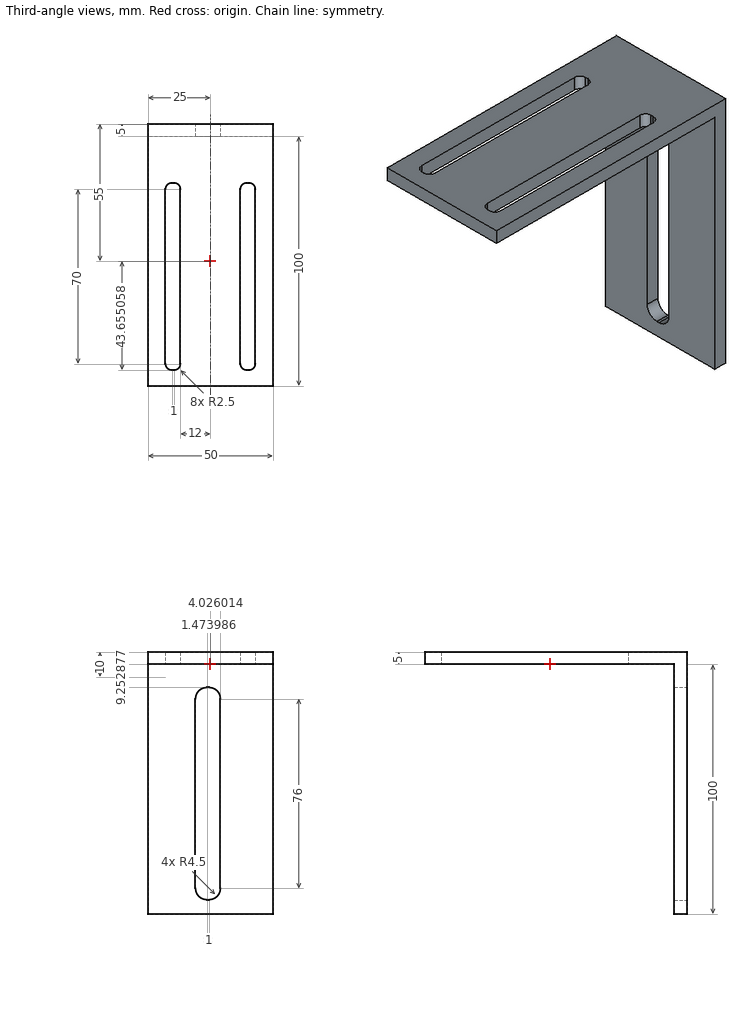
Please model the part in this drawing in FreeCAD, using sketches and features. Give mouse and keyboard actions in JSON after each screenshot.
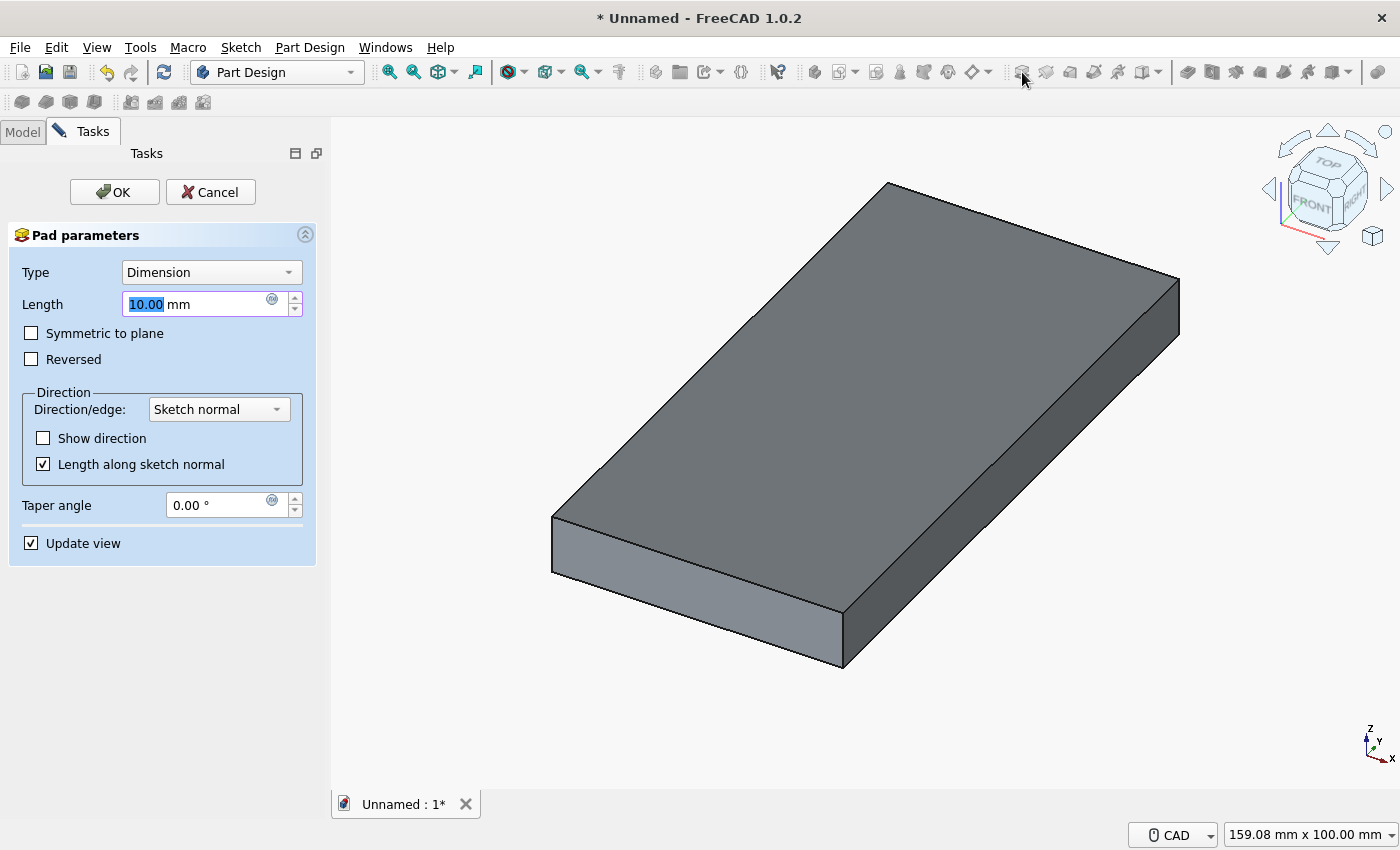
{"action": "type", "text": "5"}
{"action": "key", "text": "Tab"}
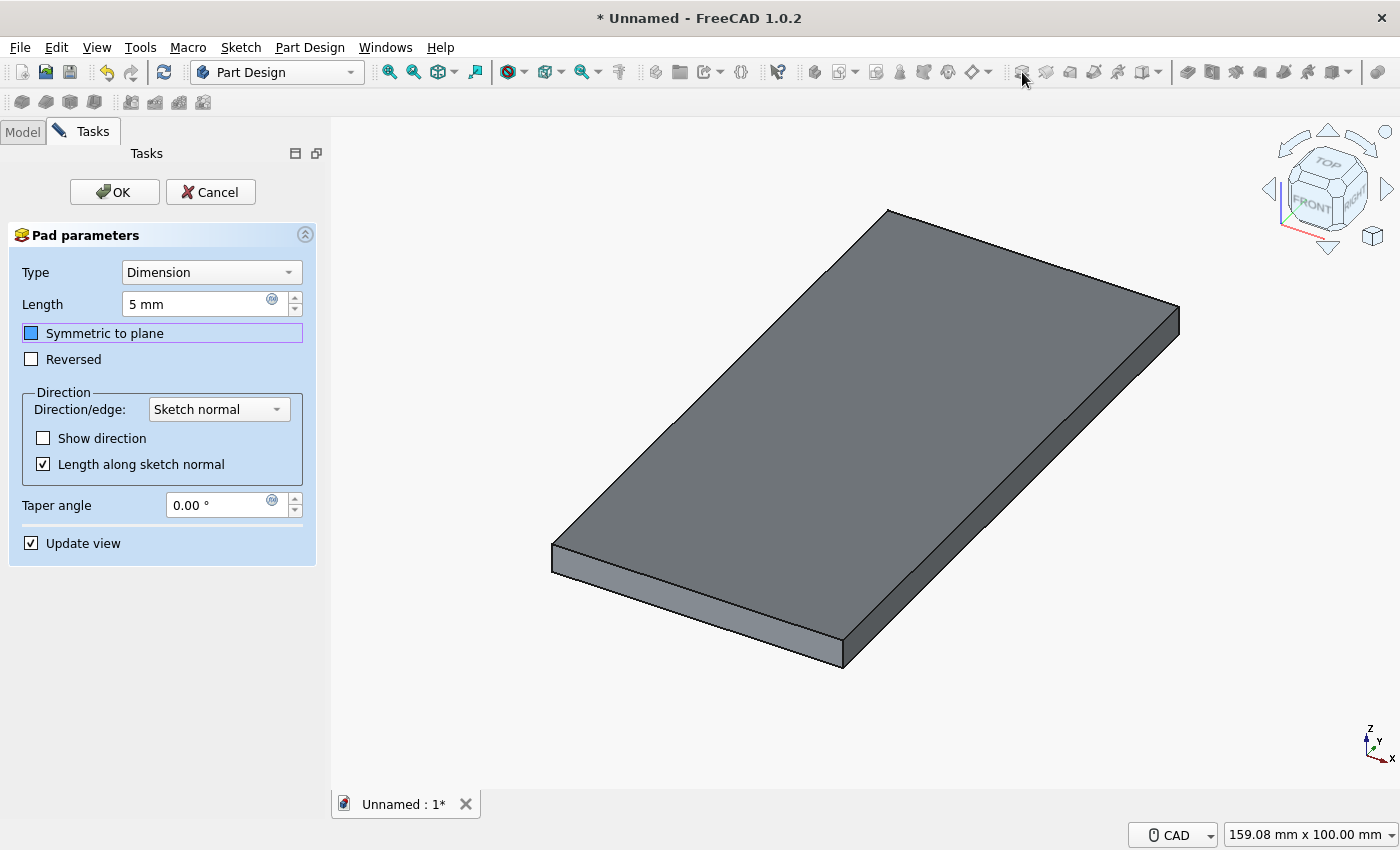
{"action": "left_click", "coordinate": [115, 192]}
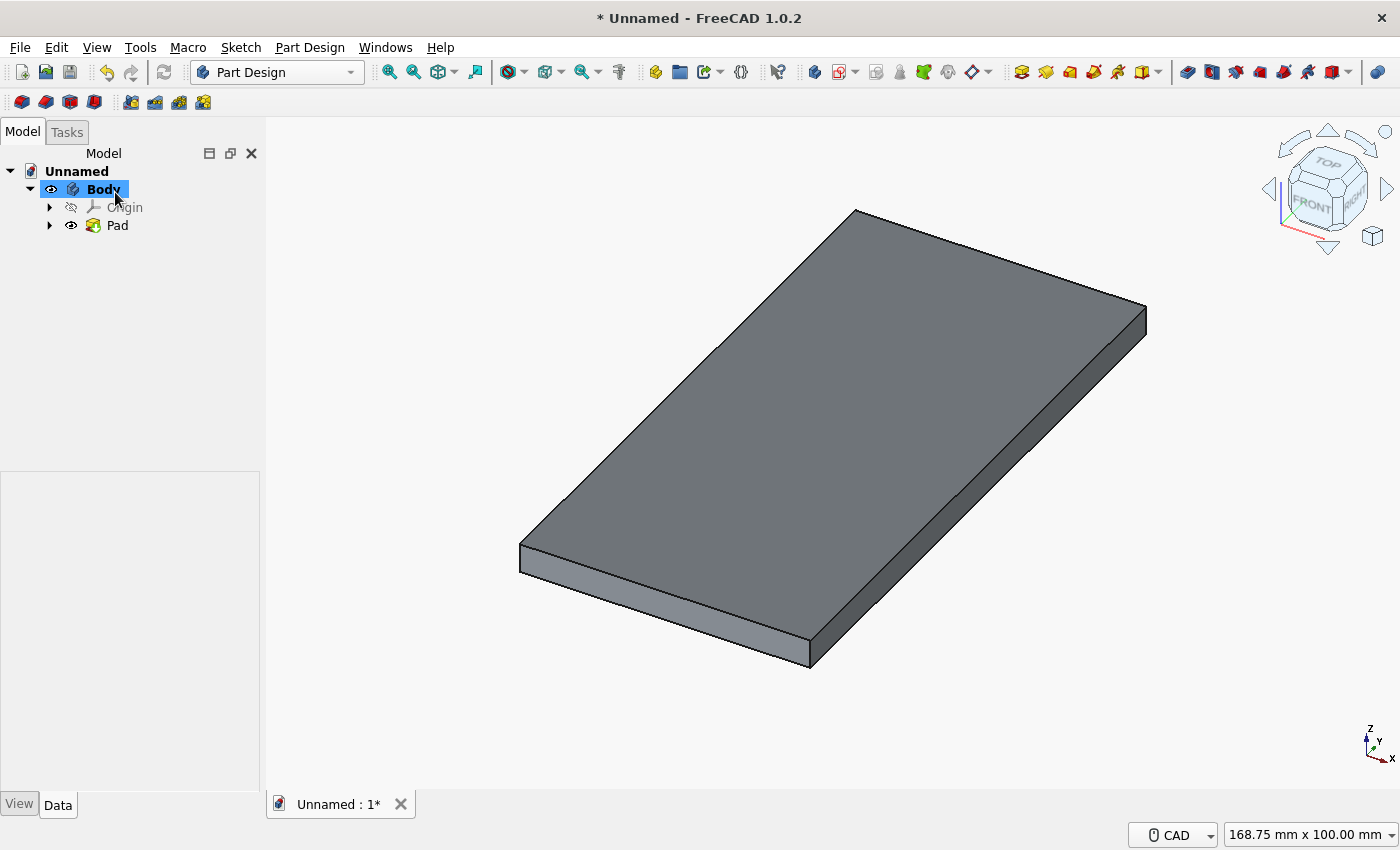
{"action": "left_click", "coordinate": [881, 377]}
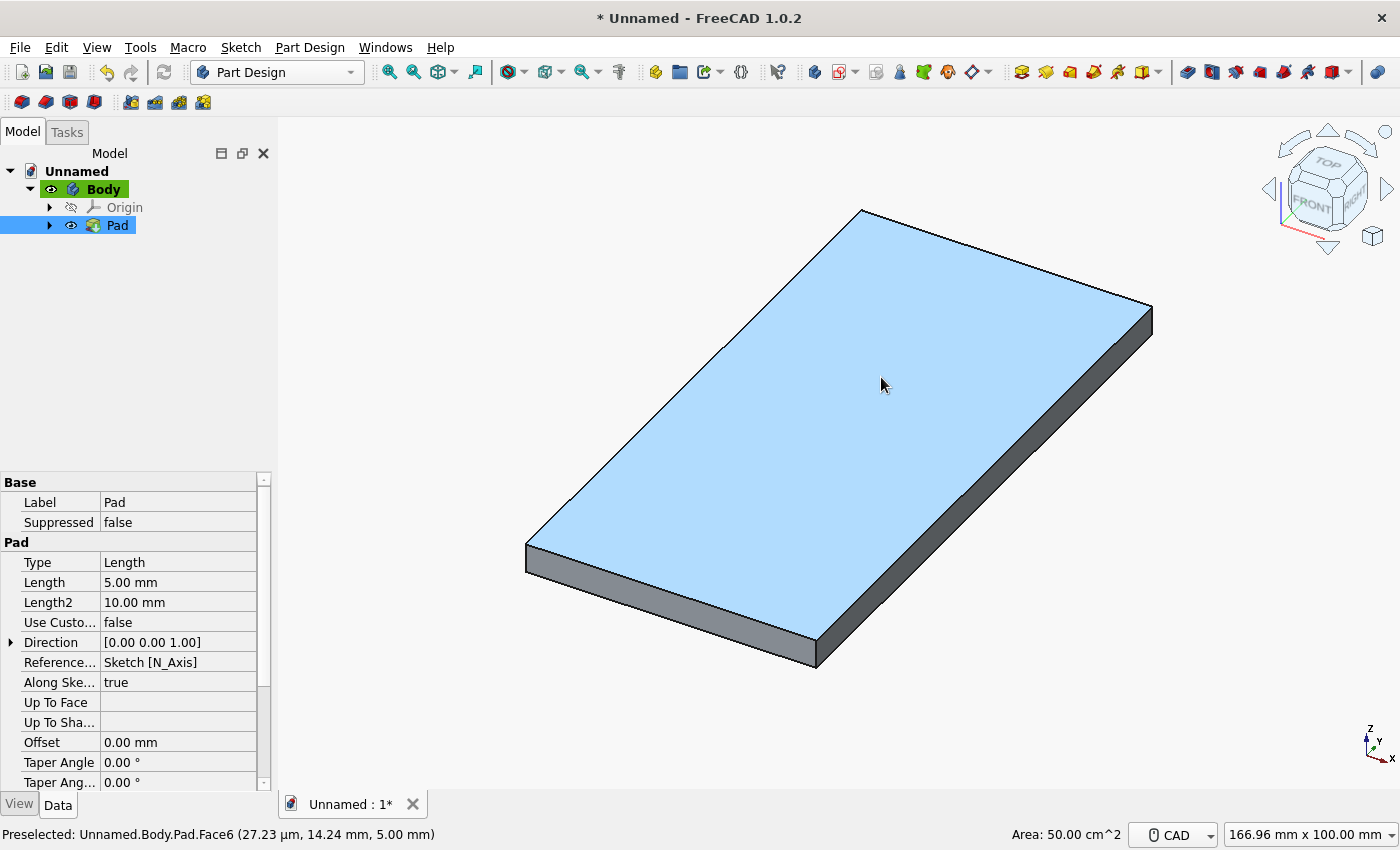
{"action": "left_click", "coordinate": [840, 72]}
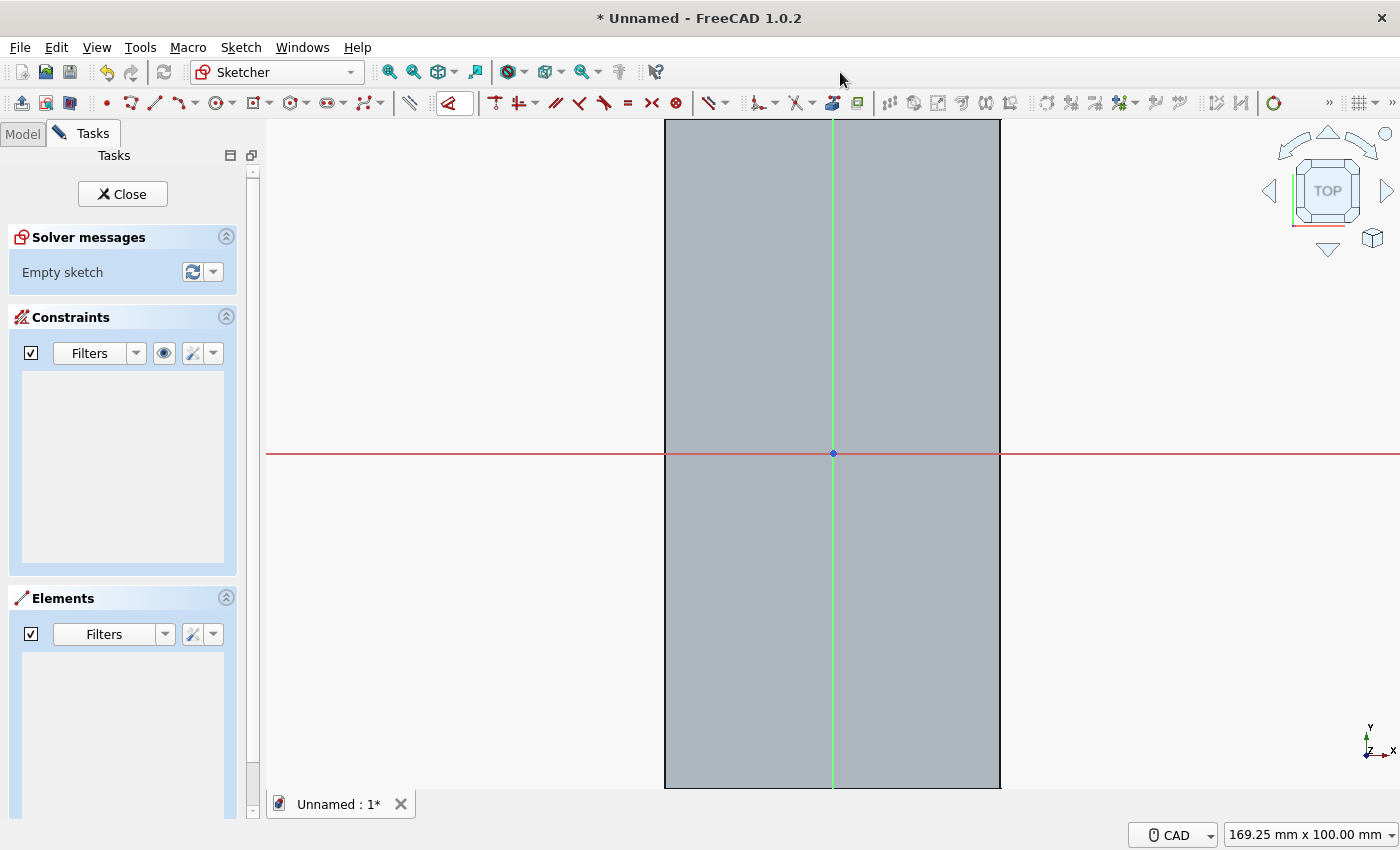
{"action": "scroll", "coordinate": [455, 268], "scroll_direction": "down", "scroll_amount": 1}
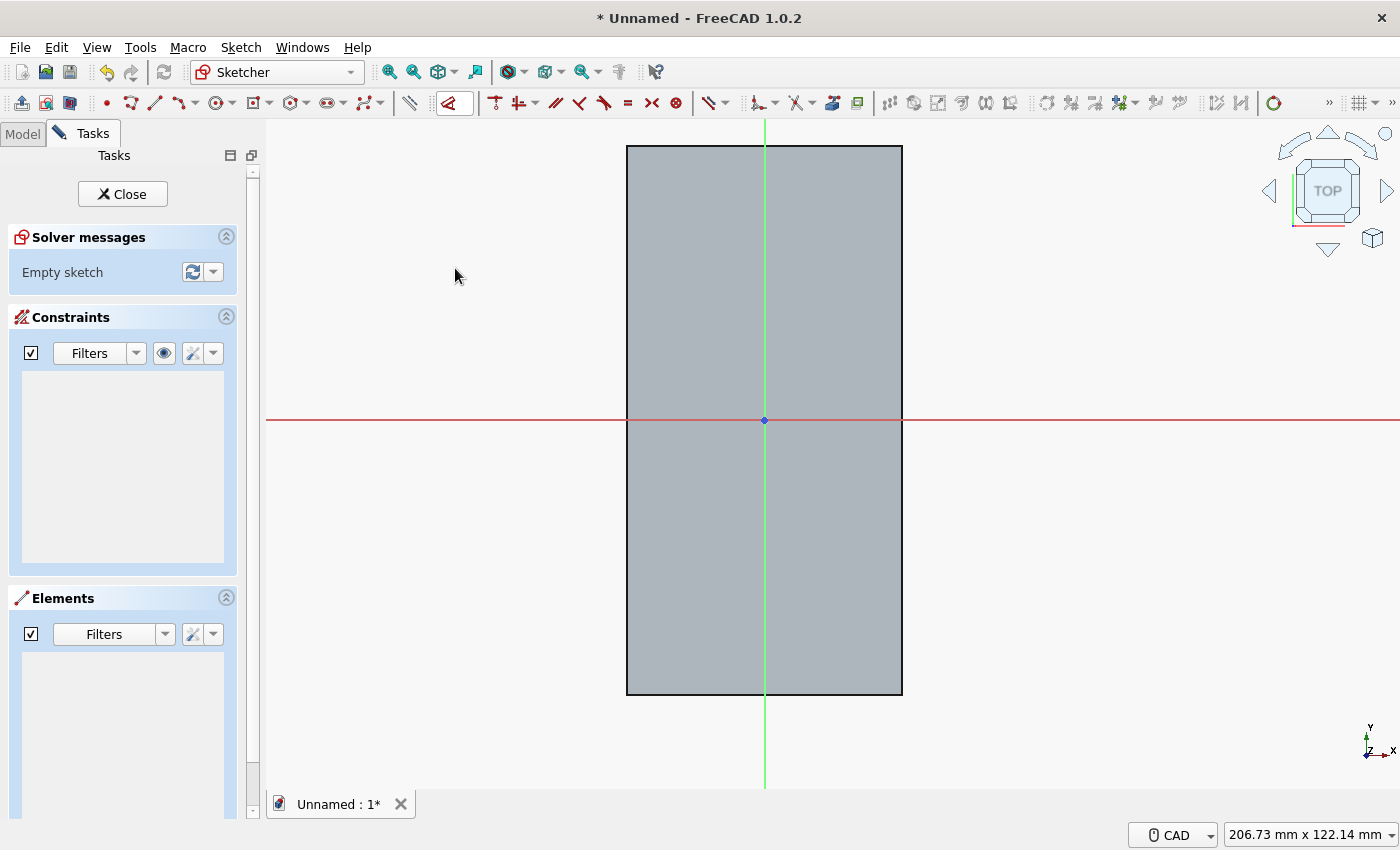
{"action": "key", "text": "g l"}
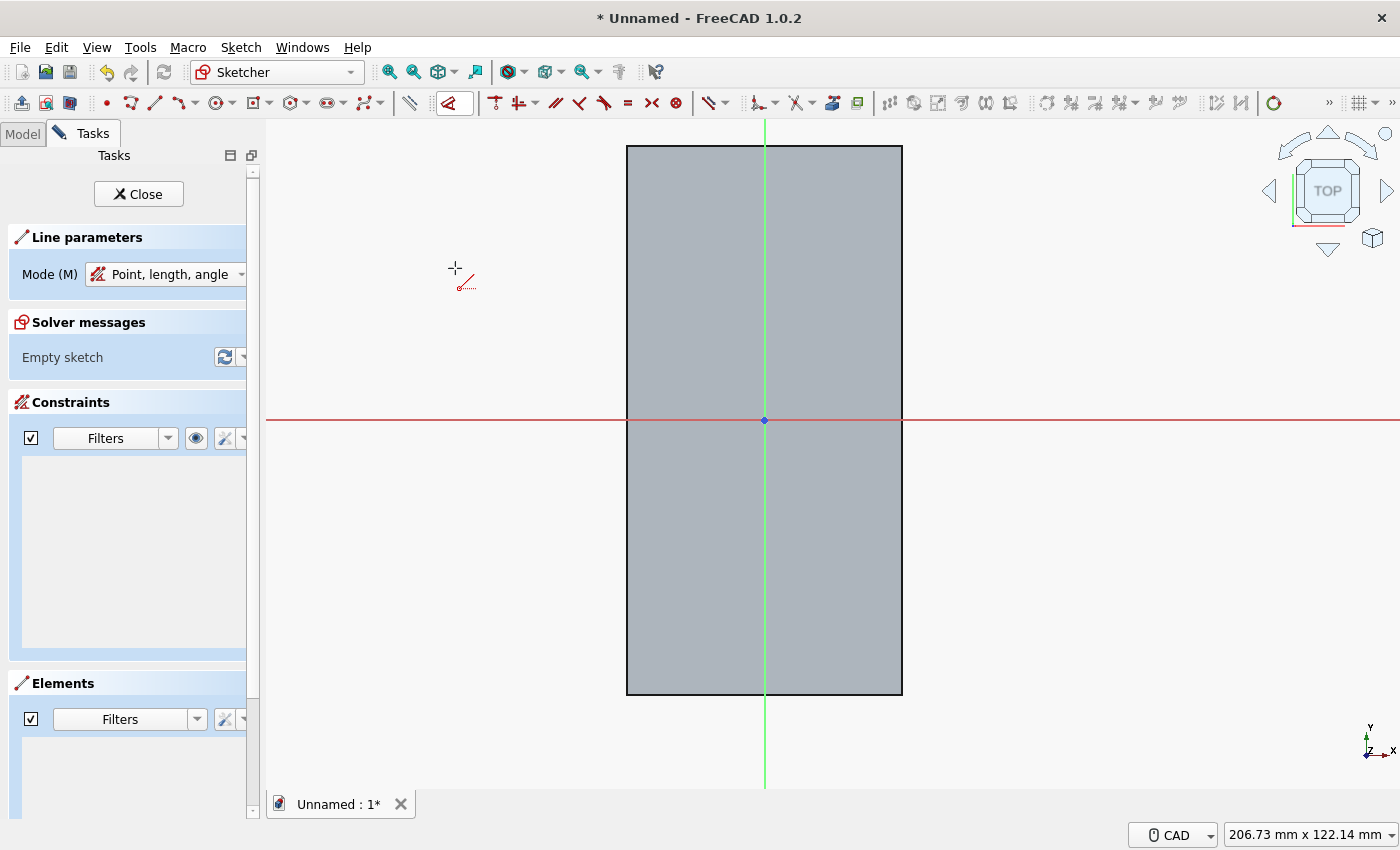
{"action": "left_click", "coordinate": [679, 660]}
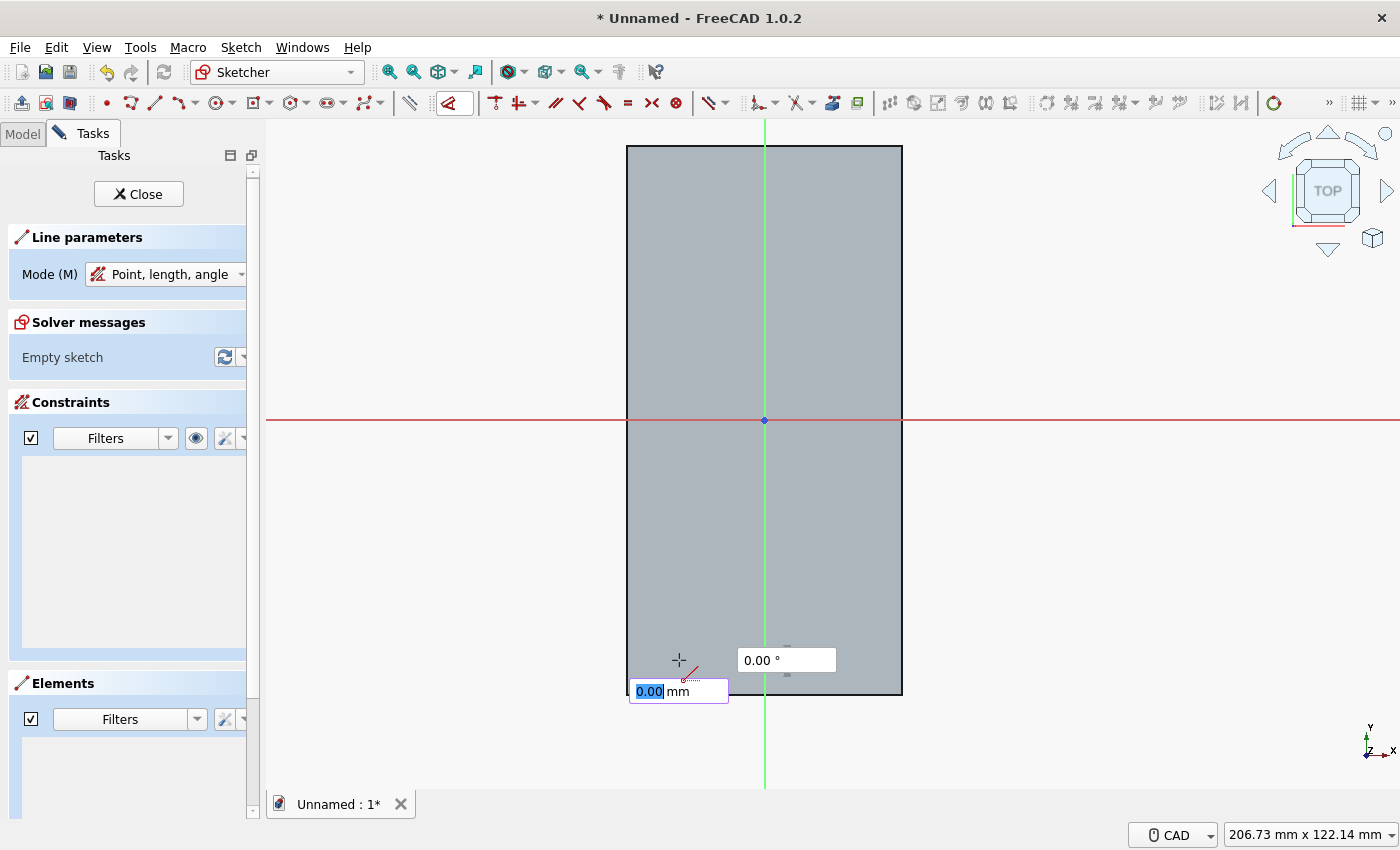
{"action": "scroll", "coordinate": [685, 660], "scroll_direction": "up", "scroll_amount": 6}